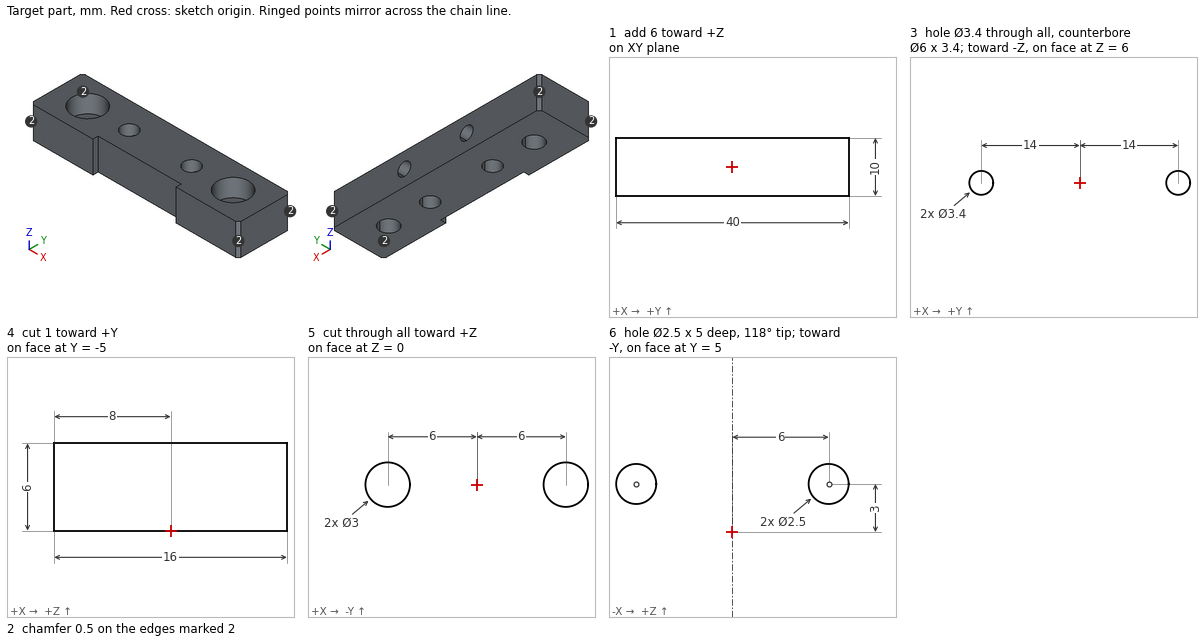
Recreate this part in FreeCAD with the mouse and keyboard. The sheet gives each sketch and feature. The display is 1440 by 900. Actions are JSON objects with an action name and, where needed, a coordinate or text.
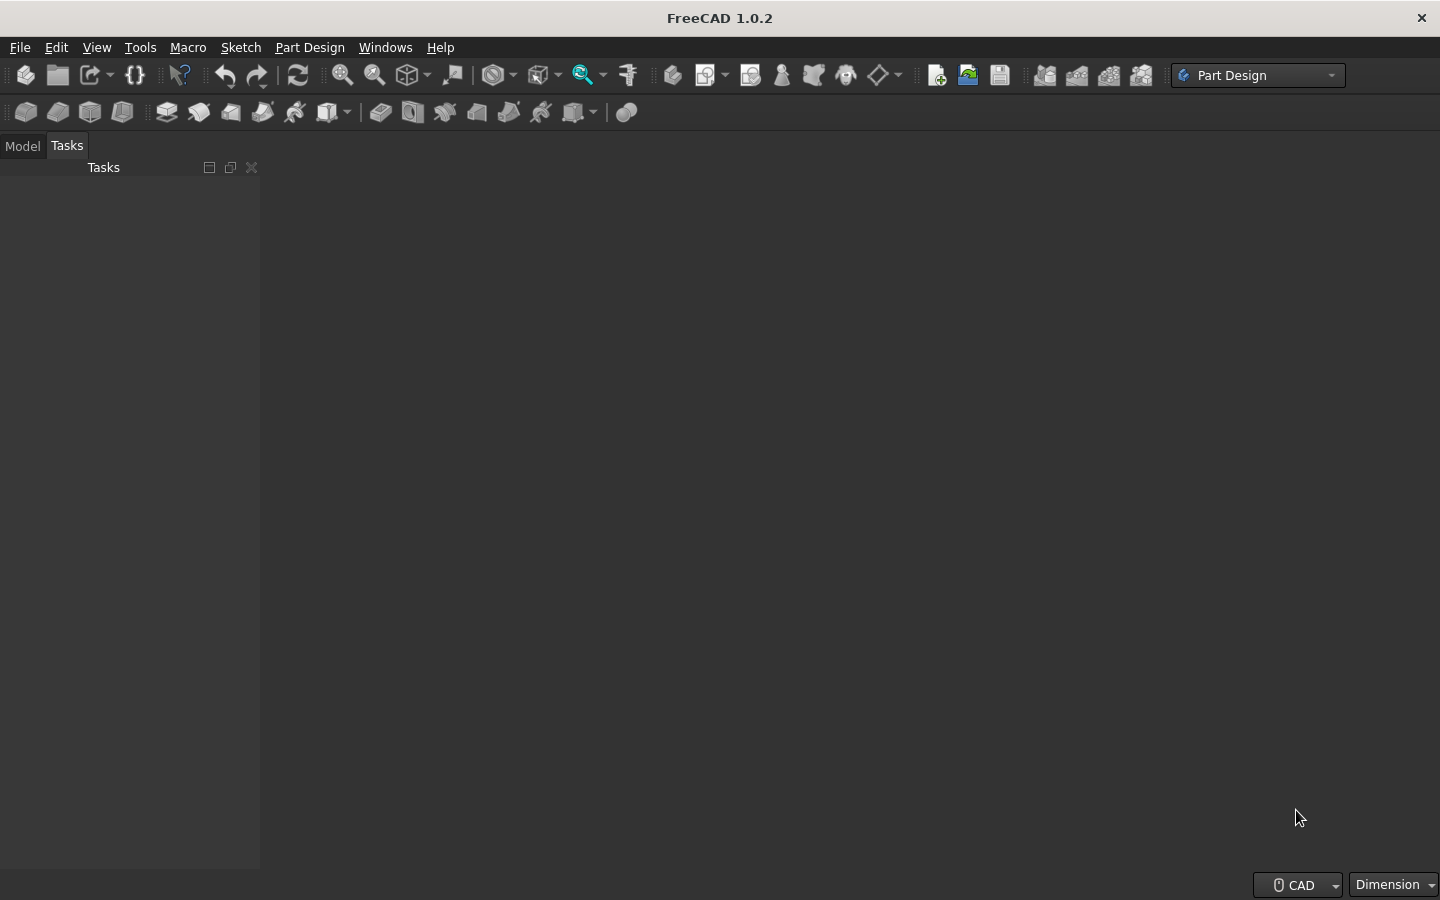
{"action": "left_click", "coordinate": [936, 76]}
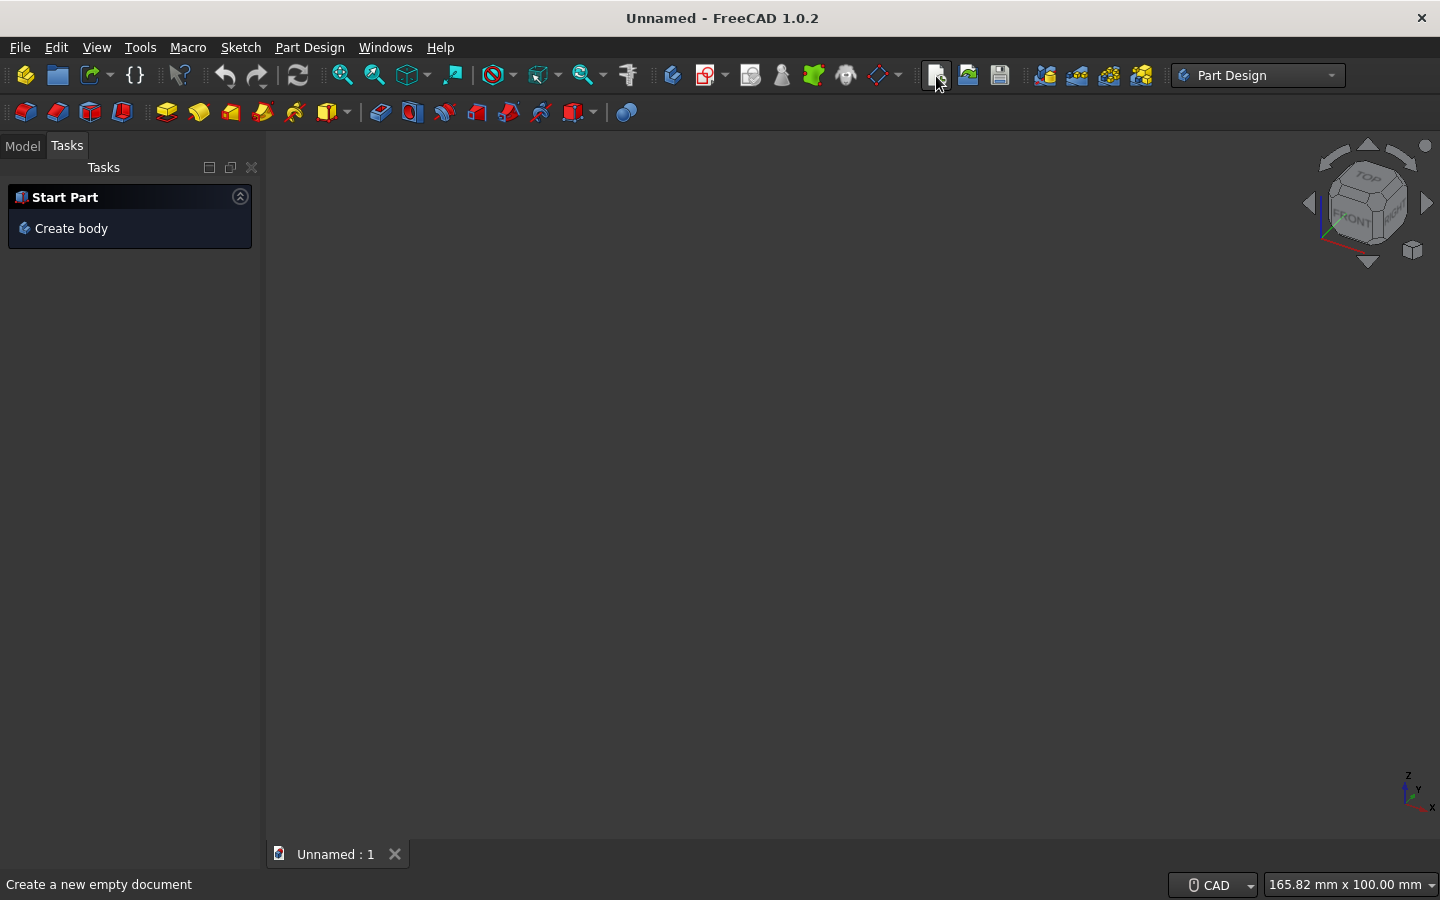
{"action": "left_click", "coordinate": [706, 76]}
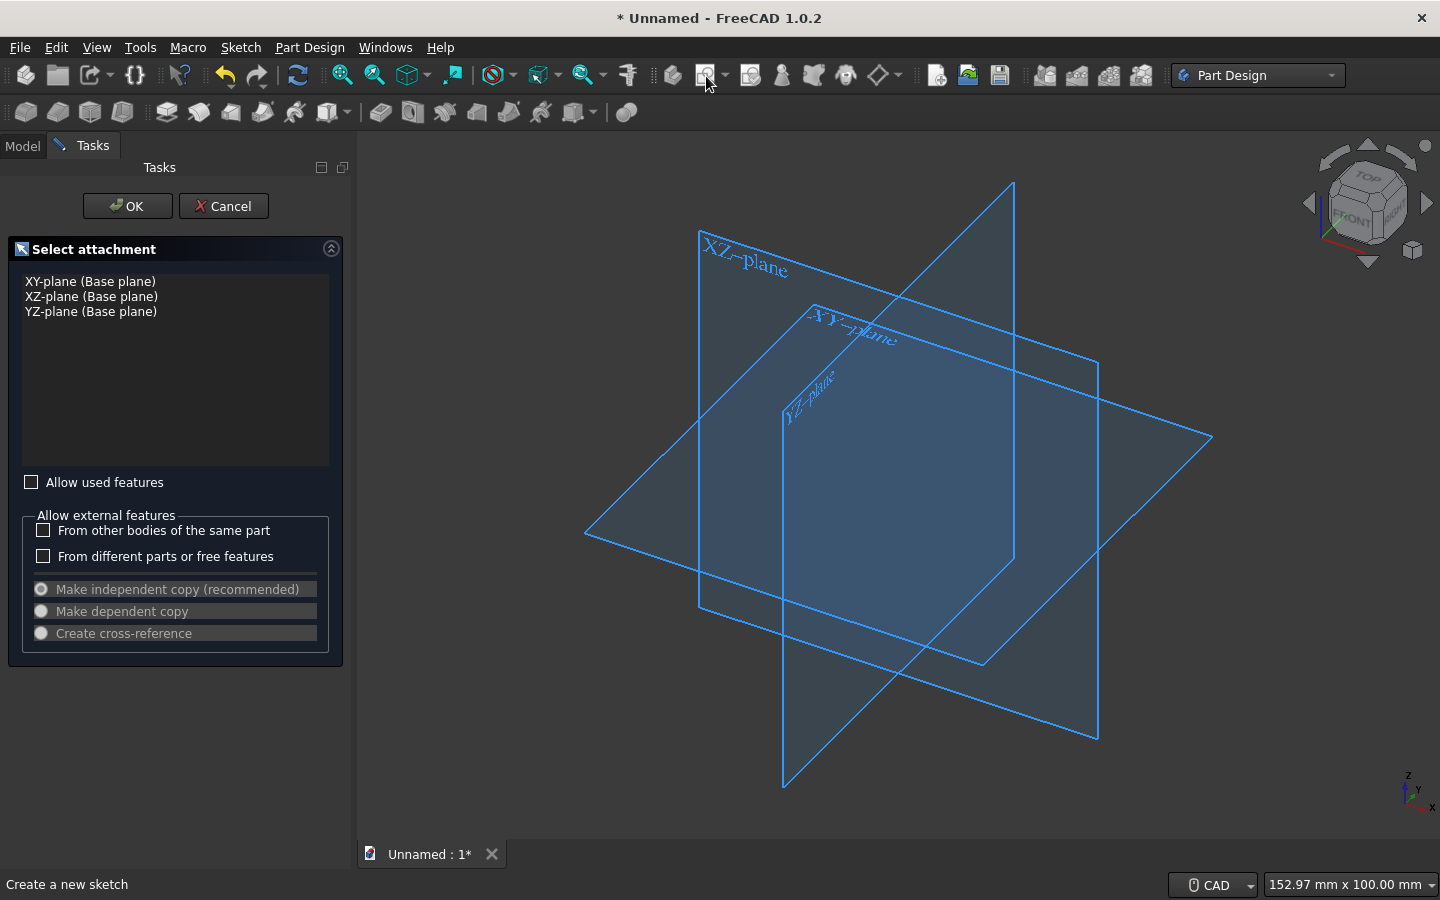
{"action": "left_click", "coordinate": [82, 282]}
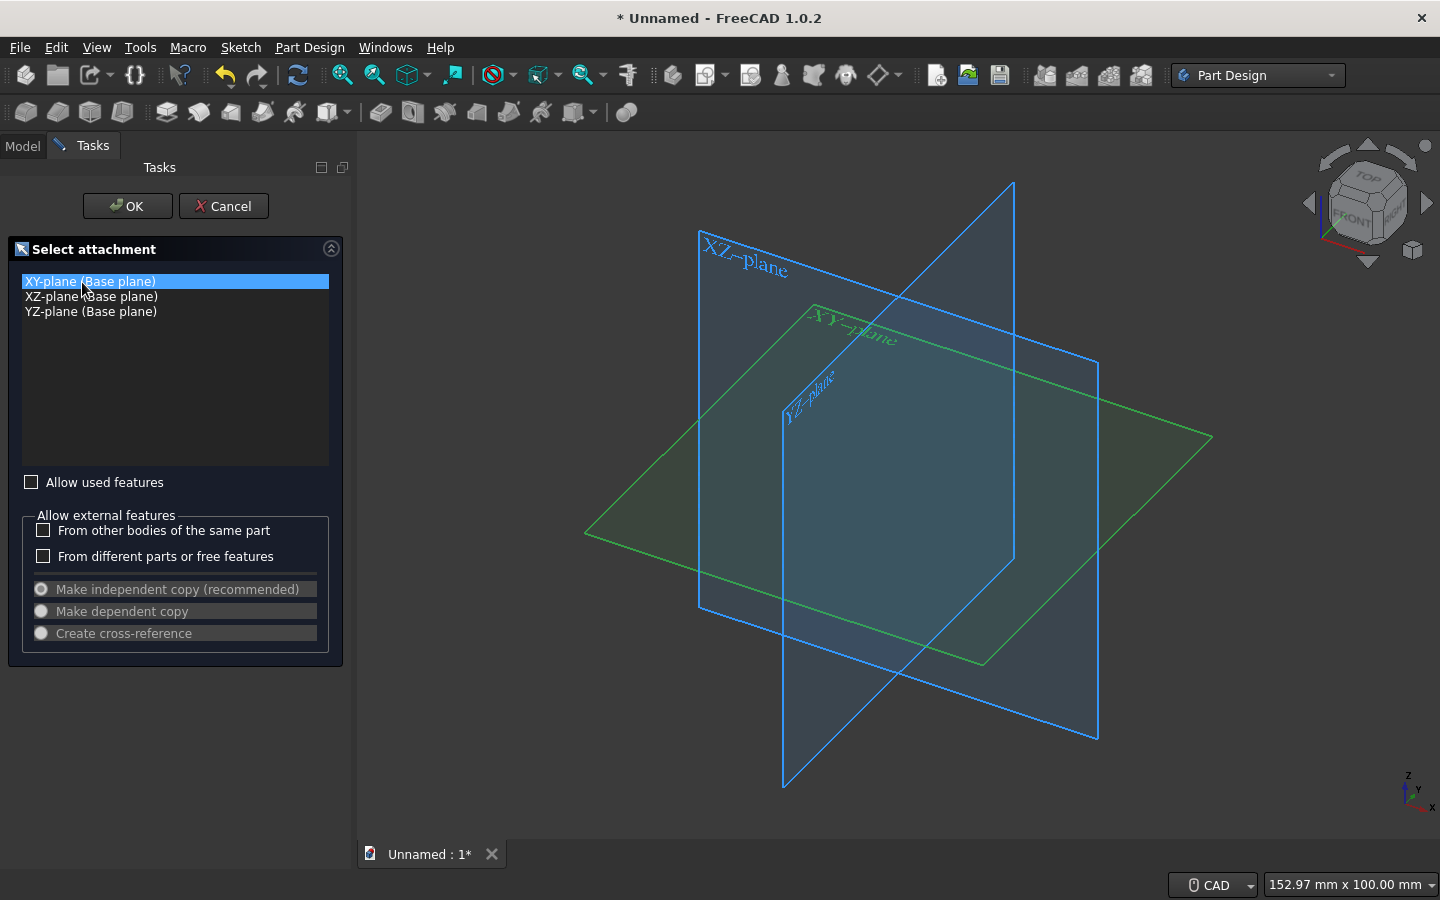
{"action": "left_click", "coordinate": [128, 206]}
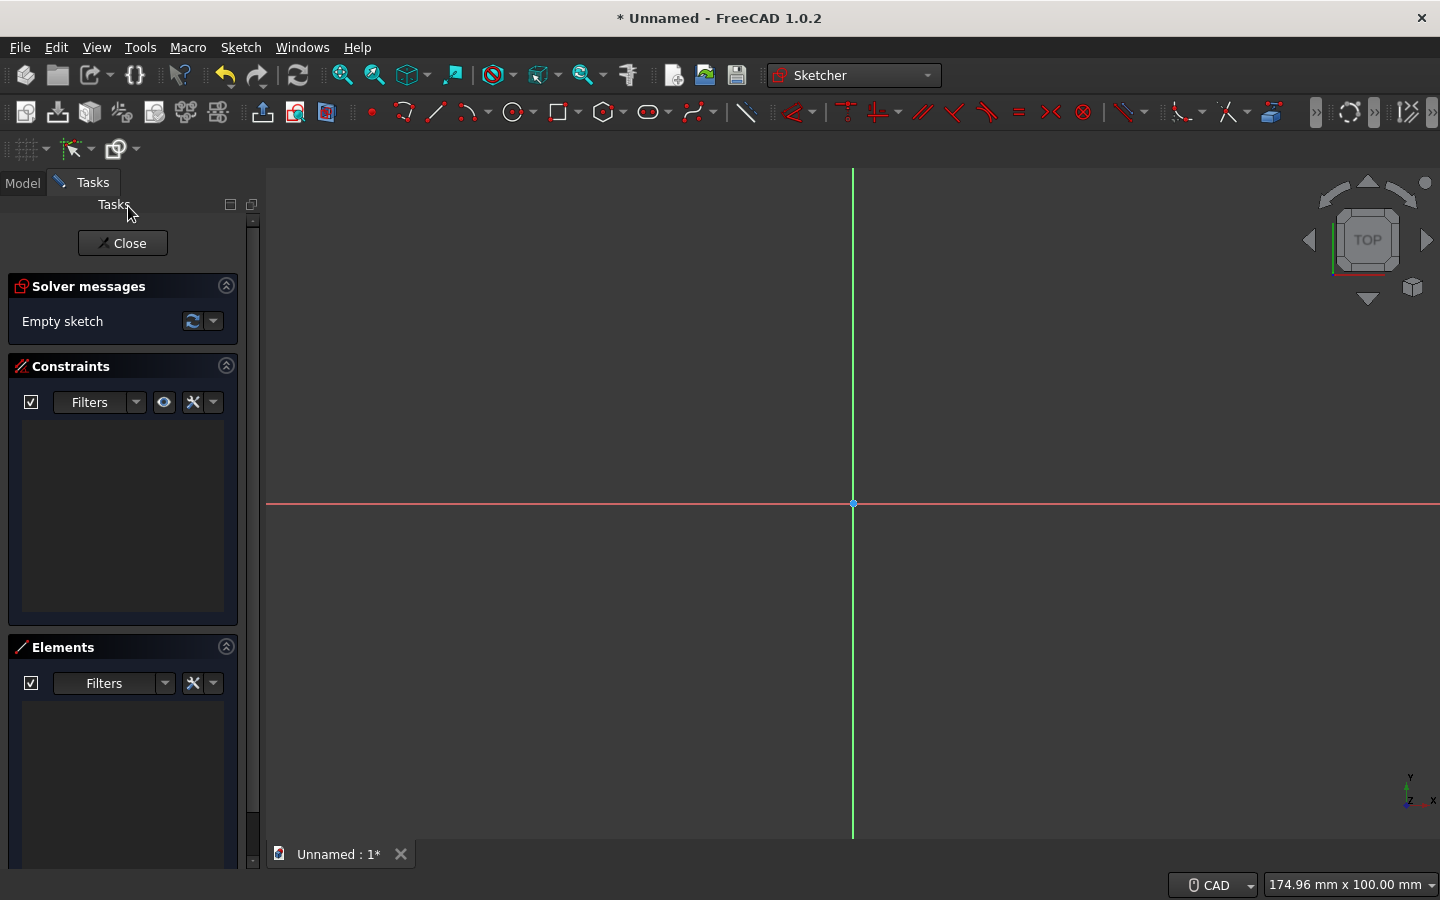
{"action": "scroll", "coordinate": [893, 504], "scroll_direction": "up", "scroll_amount": 5}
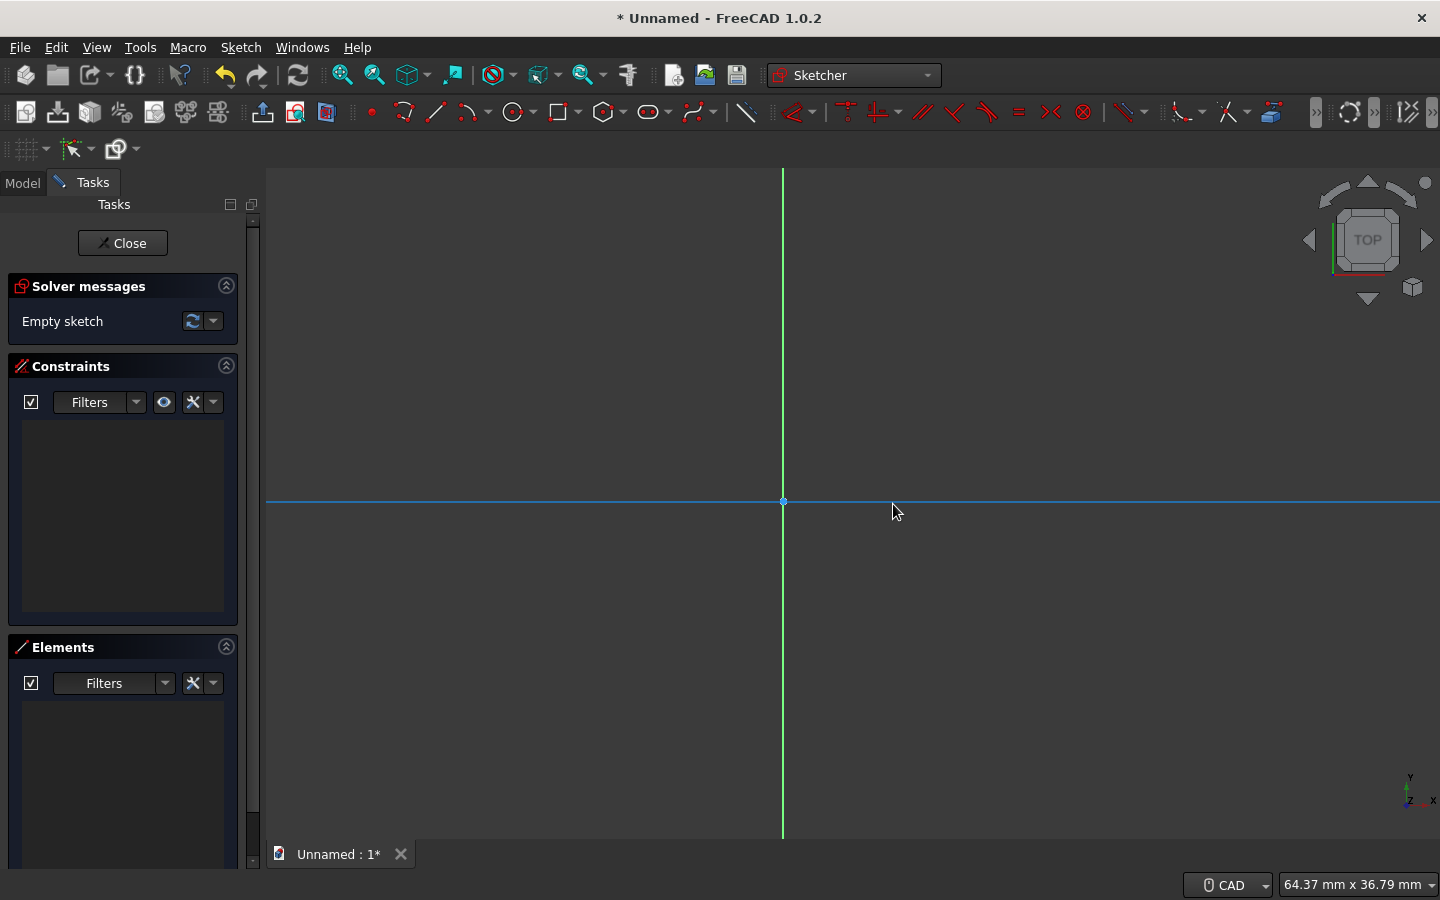
{"action": "key", "text": "g v"}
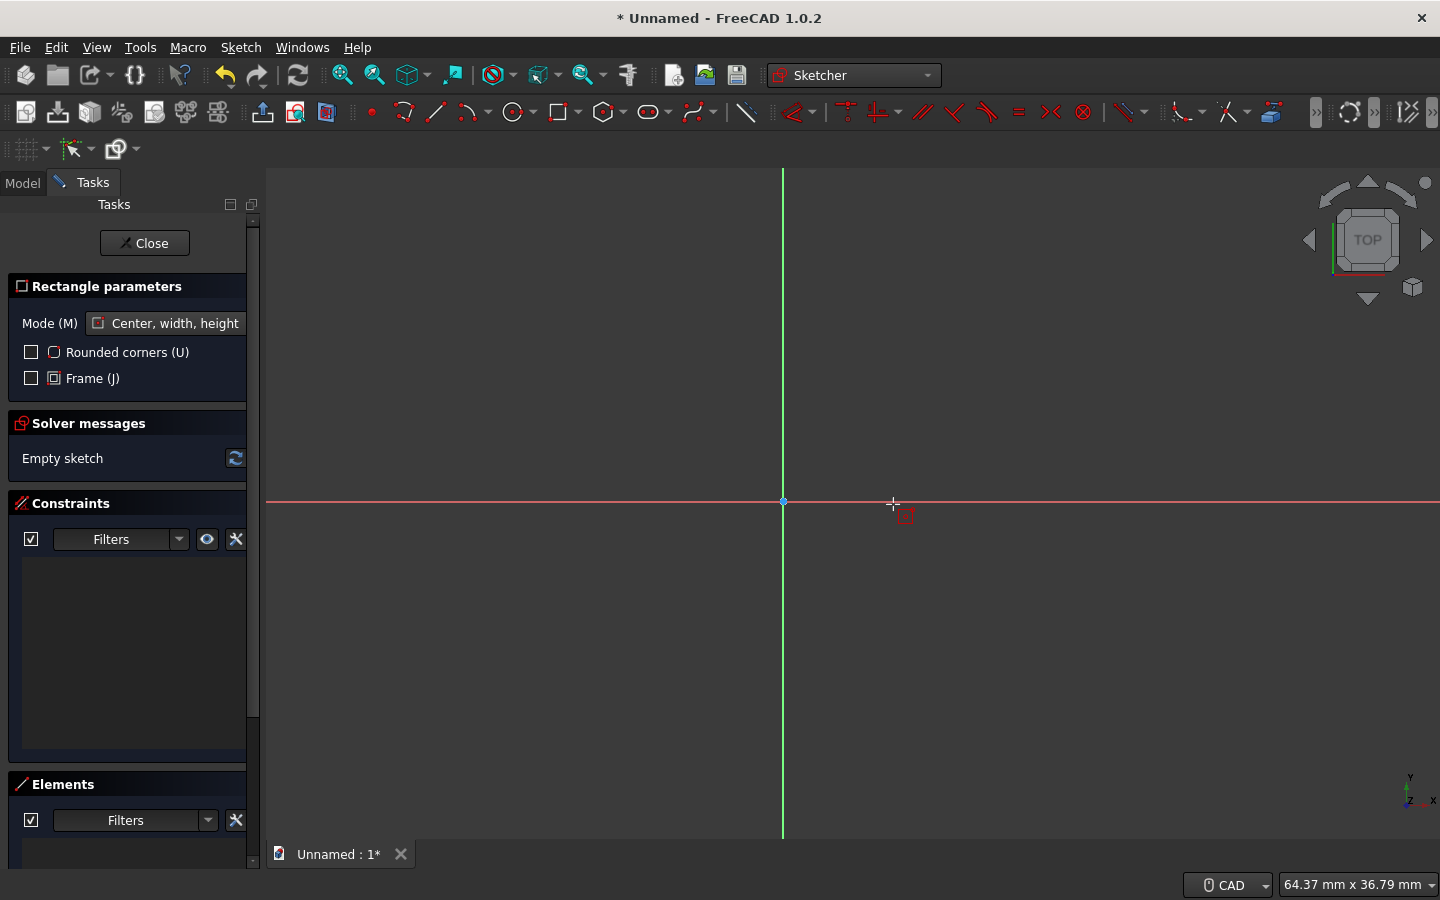
{"action": "left_click", "coordinate": [783, 502]}
{"action": "mouse_move", "coordinate": [1148, 411]}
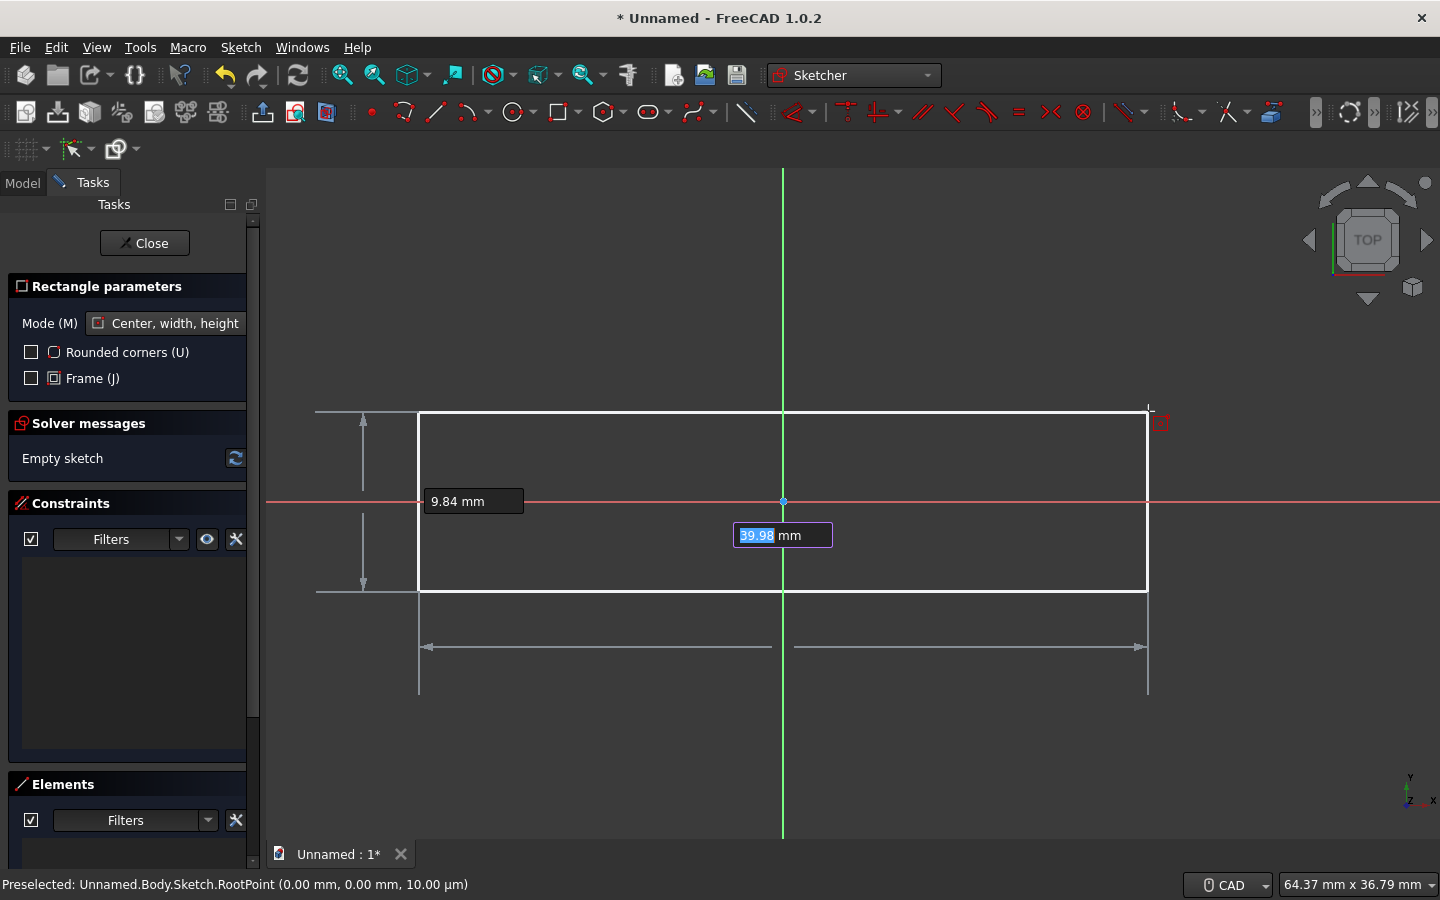
{"action": "type", "text": "40"}
{"action": "key", "text": "Tab"}
{"action": "type", "text": "10"}
{"action": "key", "text": "Return"}
{"action": "key", "text": "Escape"}